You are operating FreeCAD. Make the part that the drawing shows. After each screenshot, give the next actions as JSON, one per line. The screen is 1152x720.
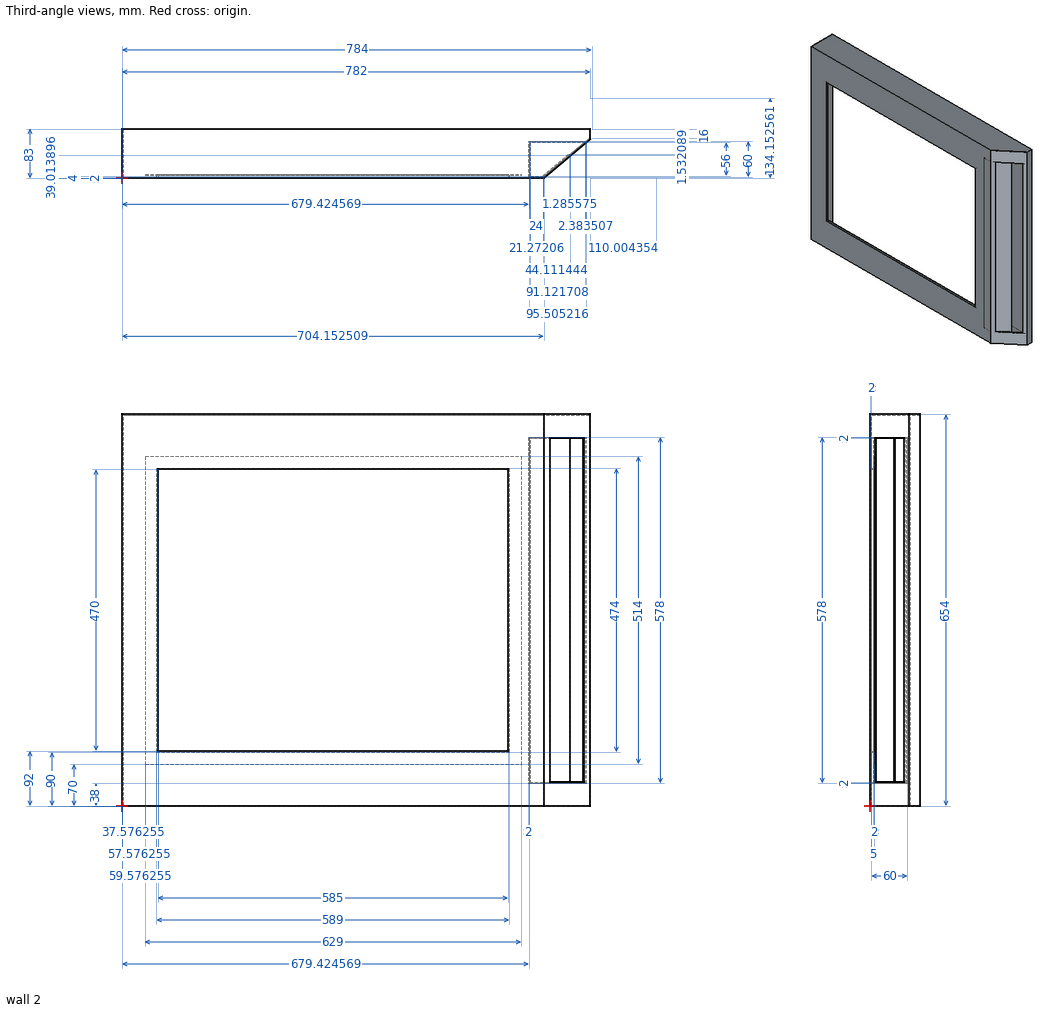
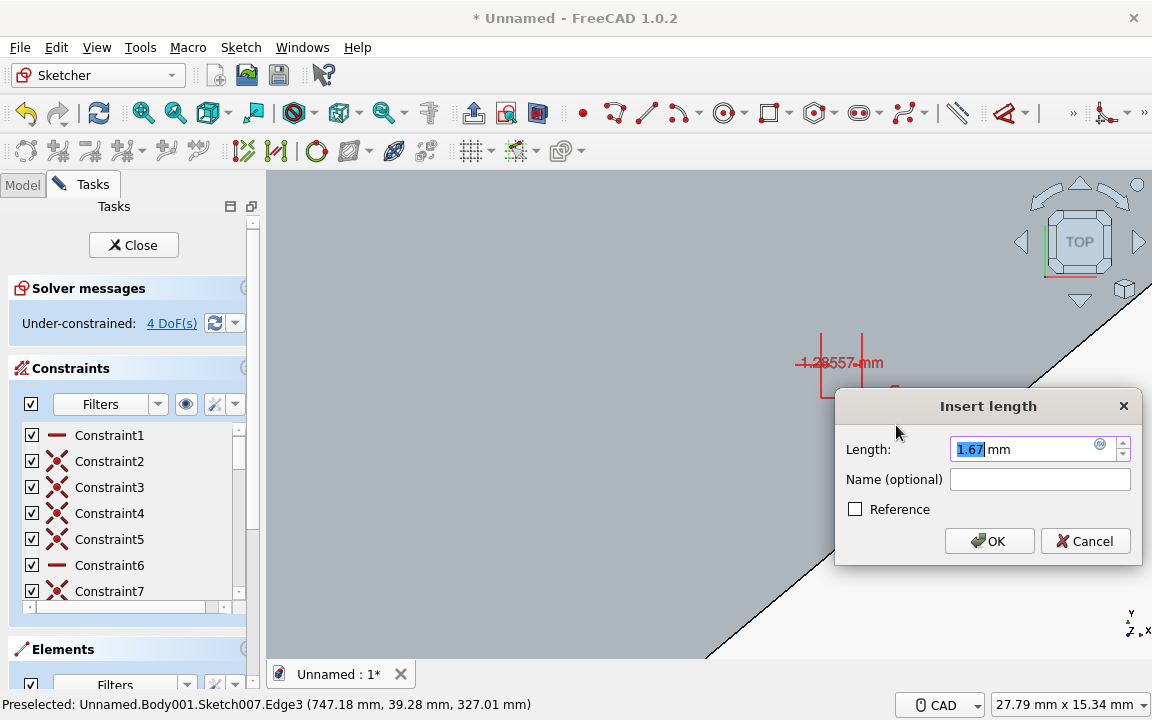
{"action": "type", "text": "1.532089"}
{"action": "key", "text": "Return"}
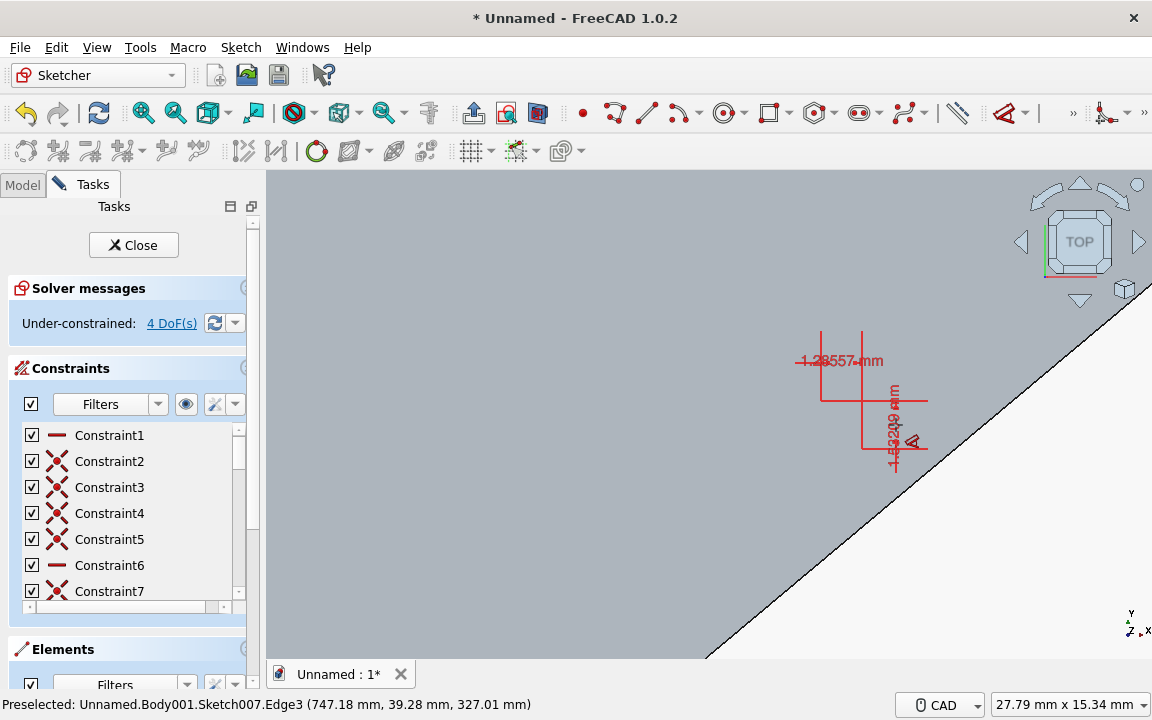
{"action": "scroll", "coordinate": [725, 364], "scroll_direction": "down", "scroll_amount": 9}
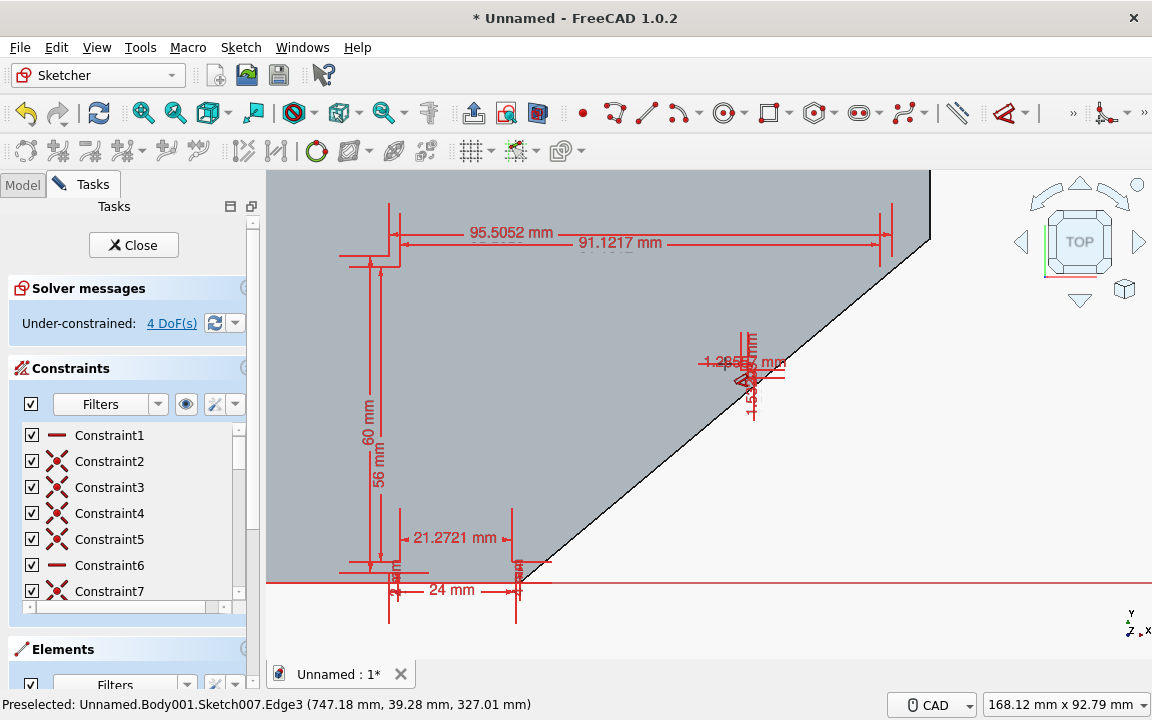
{"action": "scroll", "coordinate": [884, 264], "scroll_direction": "up", "scroll_amount": 6}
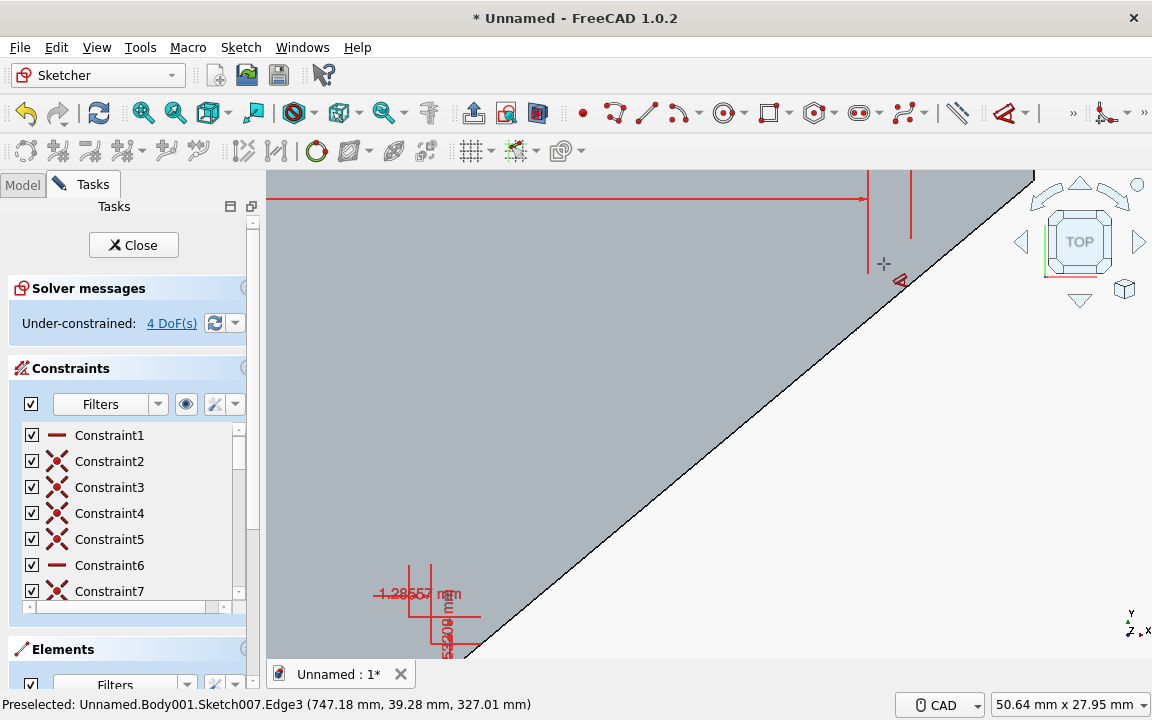
{"action": "left_click", "coordinate": [881, 263]}
{"action": "left_click", "coordinate": [889, 205]}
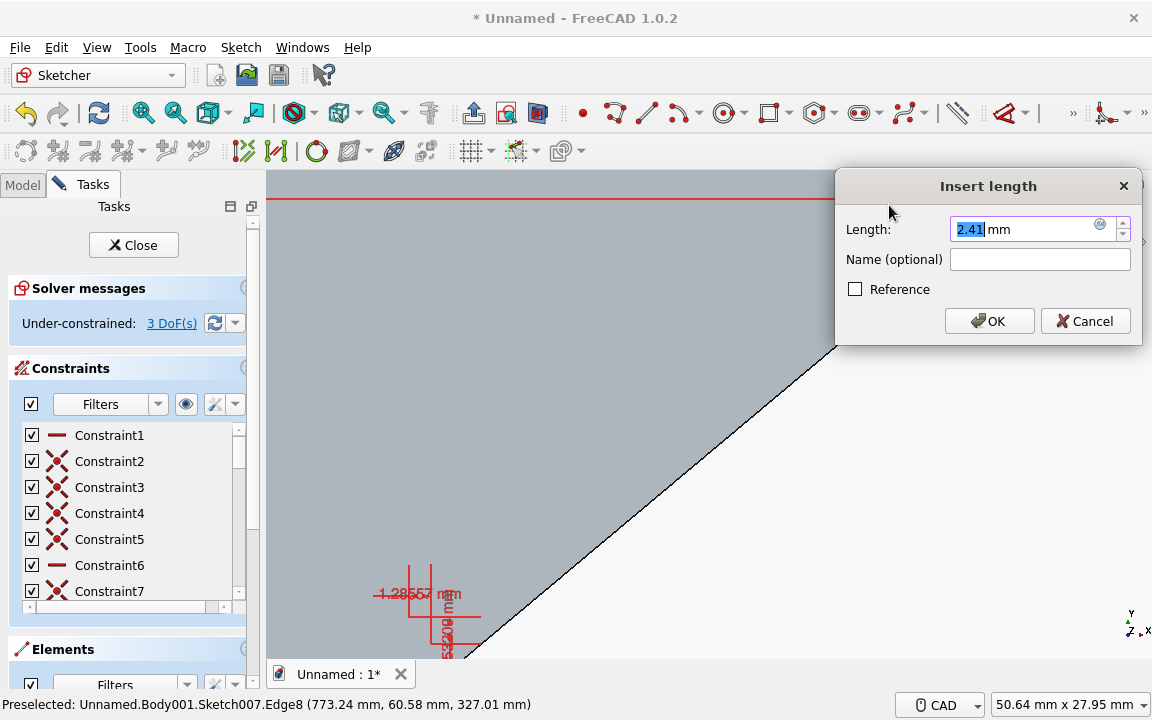
{"action": "type", "text": "2.383507"}
{"action": "key", "text": "Return"}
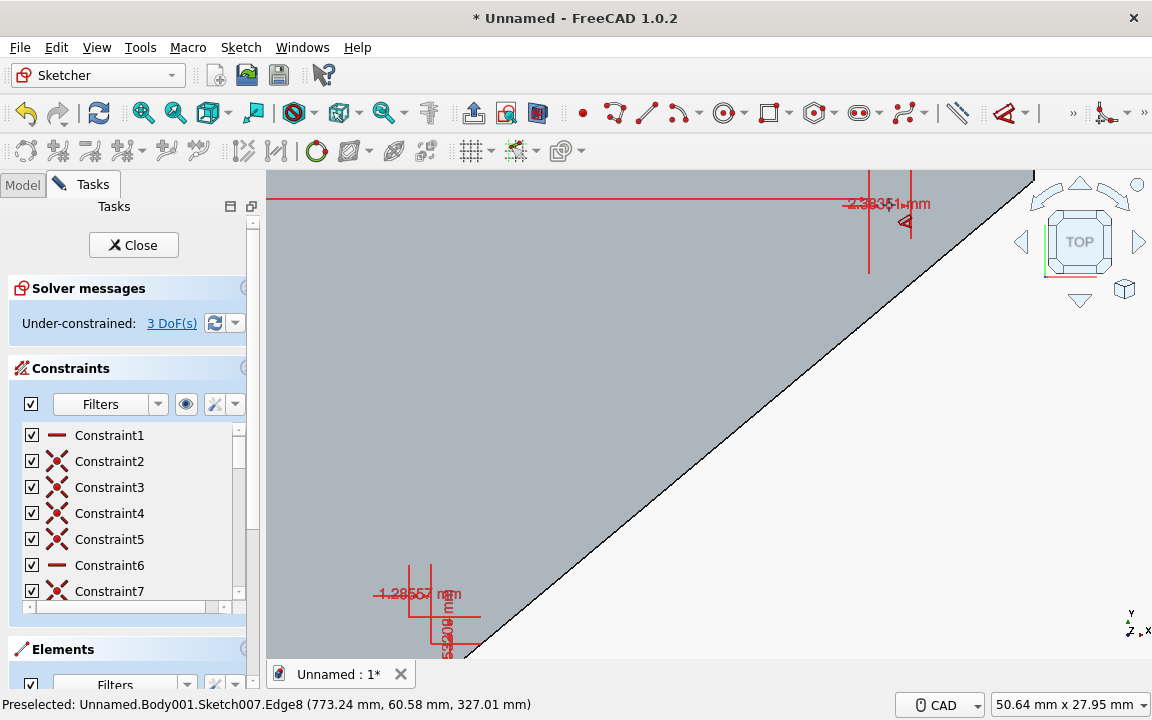
{"action": "scroll", "coordinate": [884, 264], "scroll_direction": "down", "scroll_amount": 6}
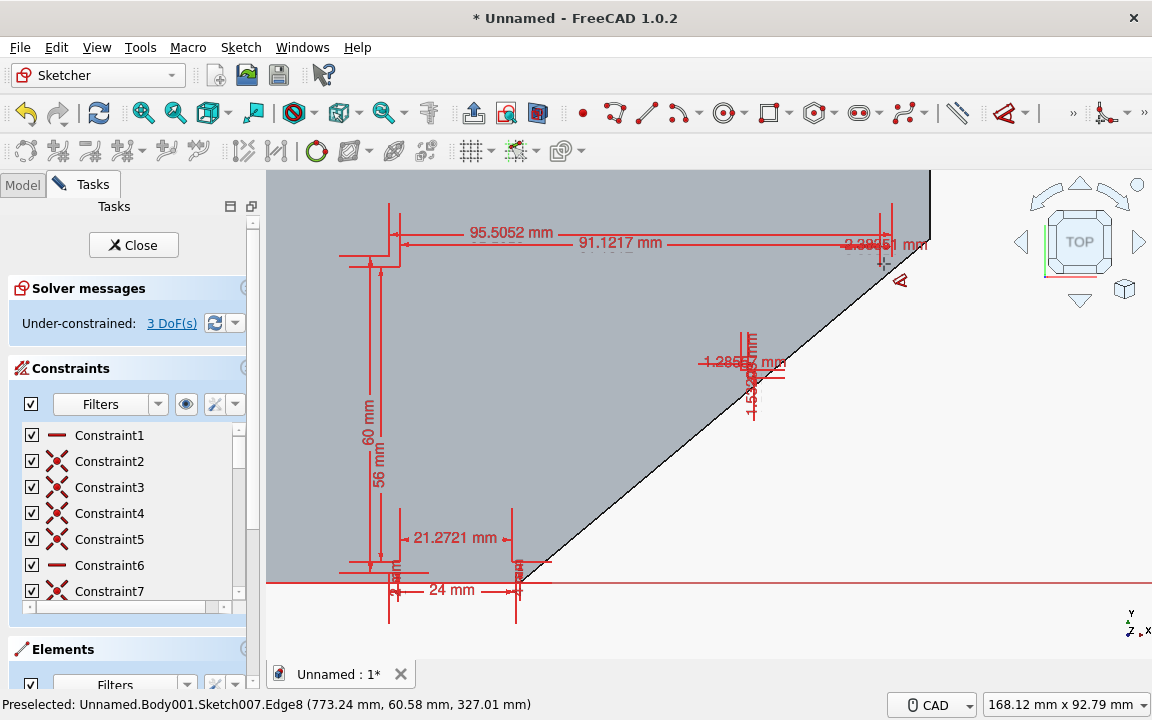
{"action": "left_click", "coordinate": [748, 378]}
{"action": "left_click", "coordinate": [782, 481]}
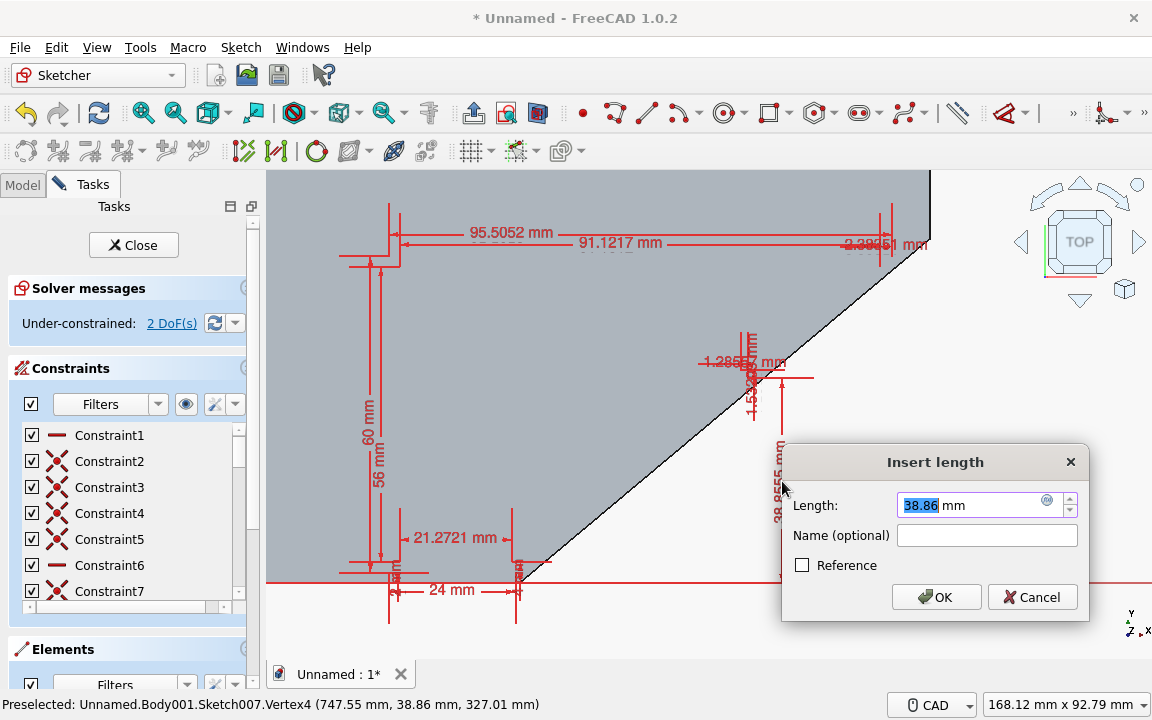
{"action": "type", "text": "39.013896"}
{"action": "key", "text": "Return"}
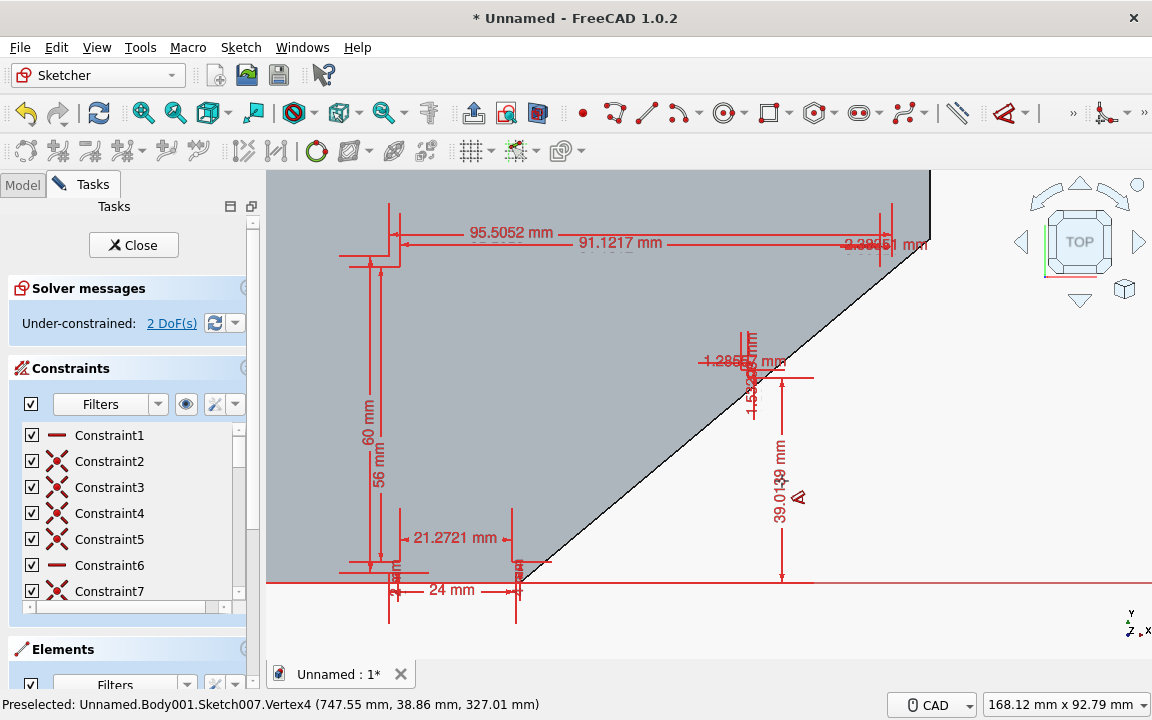
{"action": "scroll", "coordinate": [585, 514], "scroll_direction": "up", "scroll_amount": 2}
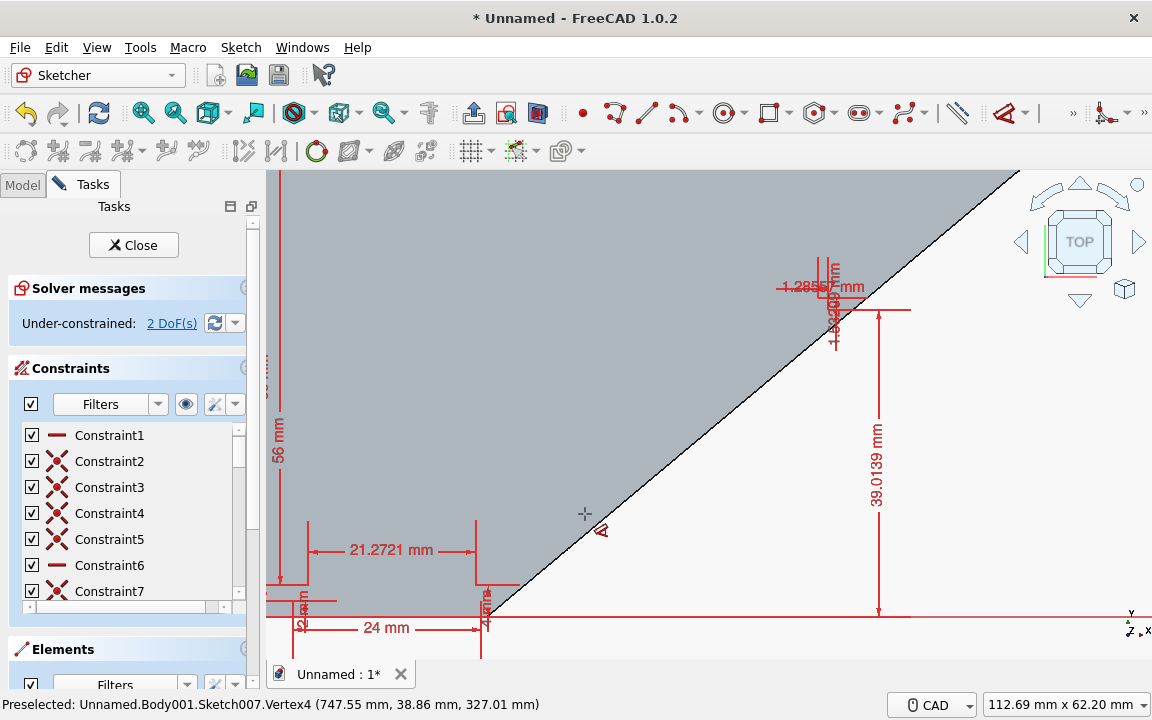
{"action": "left_click", "coordinate": [585, 514]}
{"action": "left_click", "coordinate": [655, 276]}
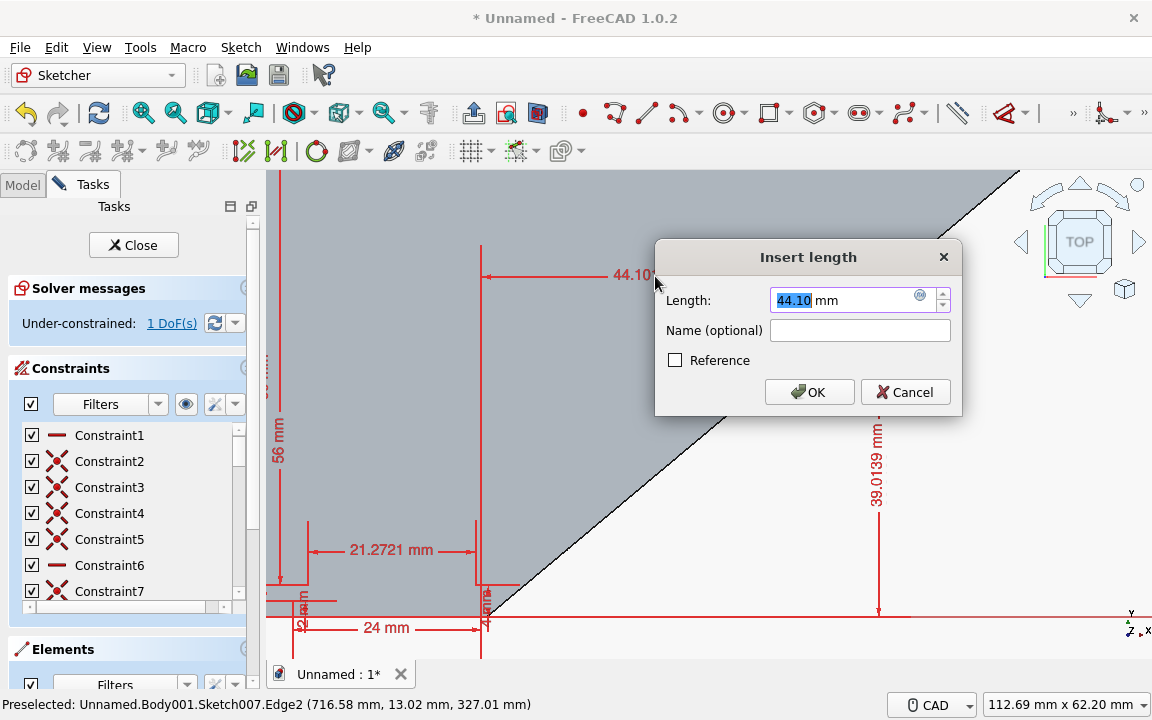
{"action": "type", "text": "44.111444"}
{"action": "key", "text": "Return"}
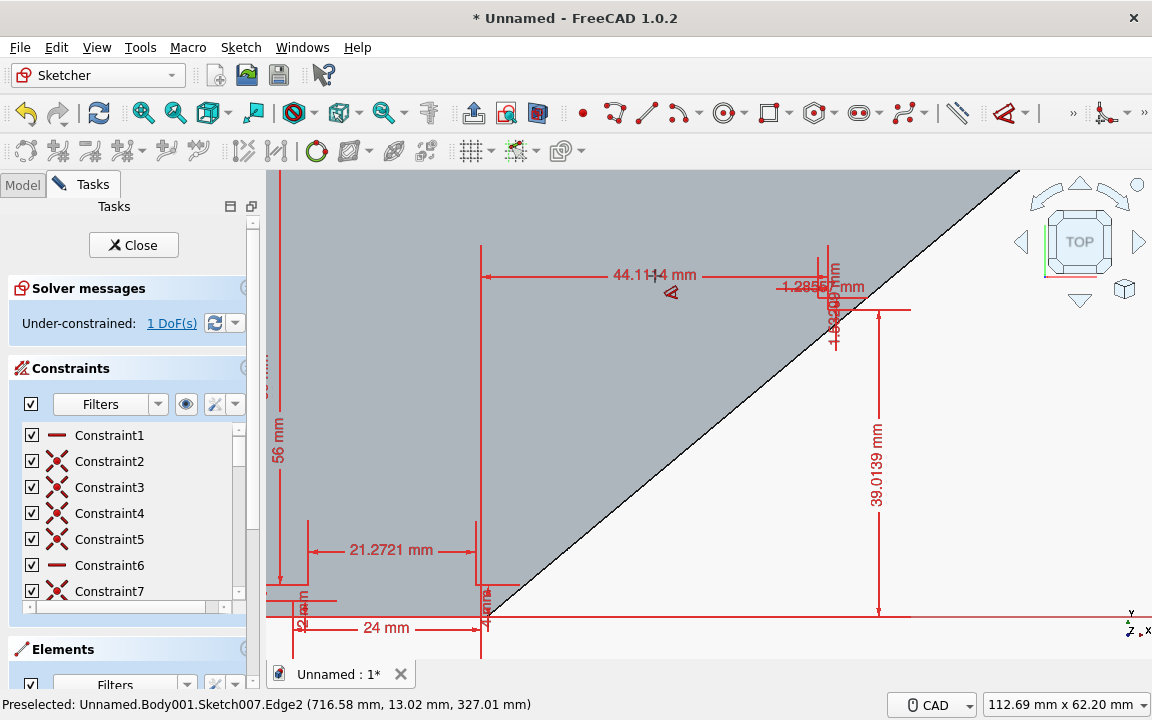
{"action": "scroll", "coordinate": [585, 514], "scroll_direction": "down", "scroll_amount": 2}